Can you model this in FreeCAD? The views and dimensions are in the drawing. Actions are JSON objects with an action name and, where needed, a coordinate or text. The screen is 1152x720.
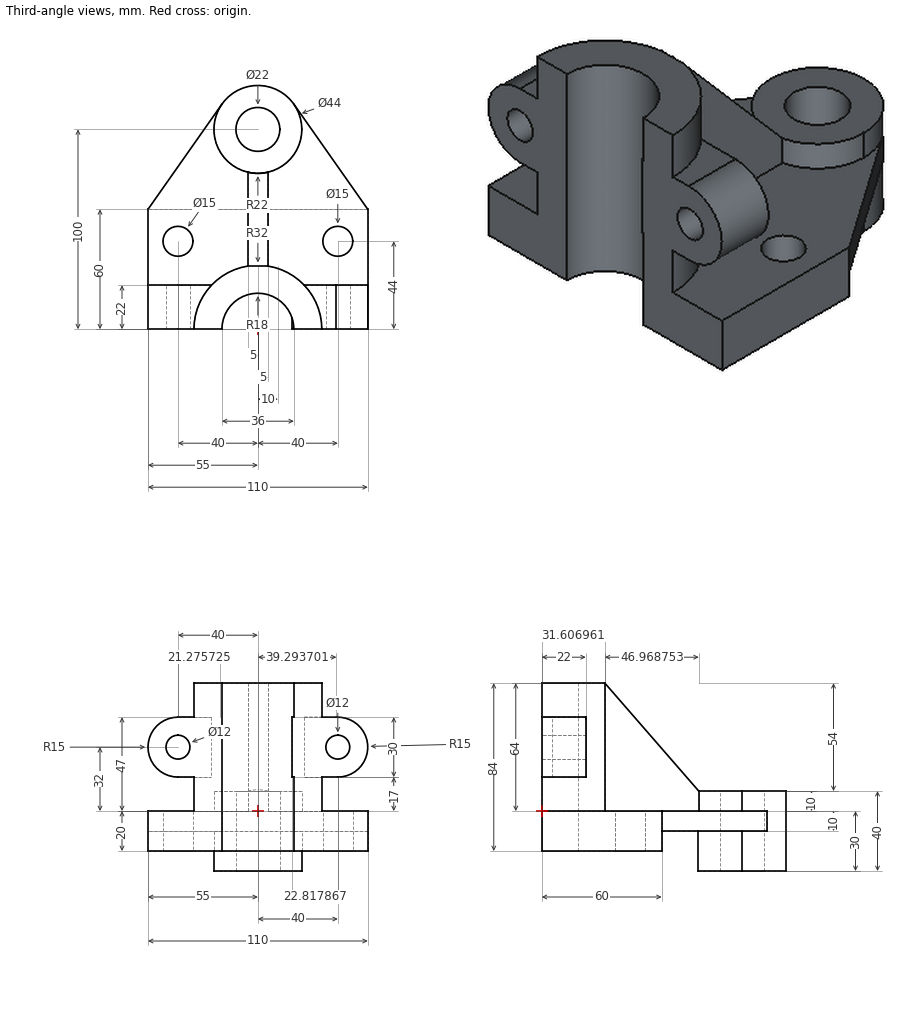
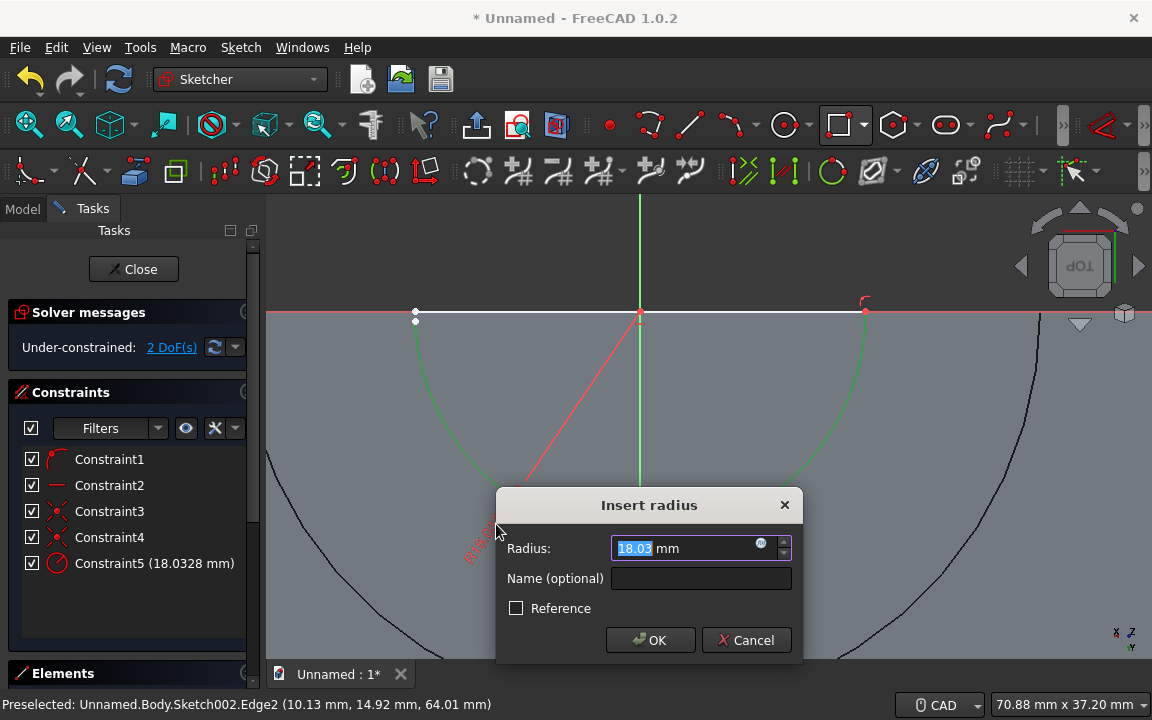
{"action": "type", "text": "18"}
{"action": "key", "text": "Return"}
{"action": "key", "text": "Escape"}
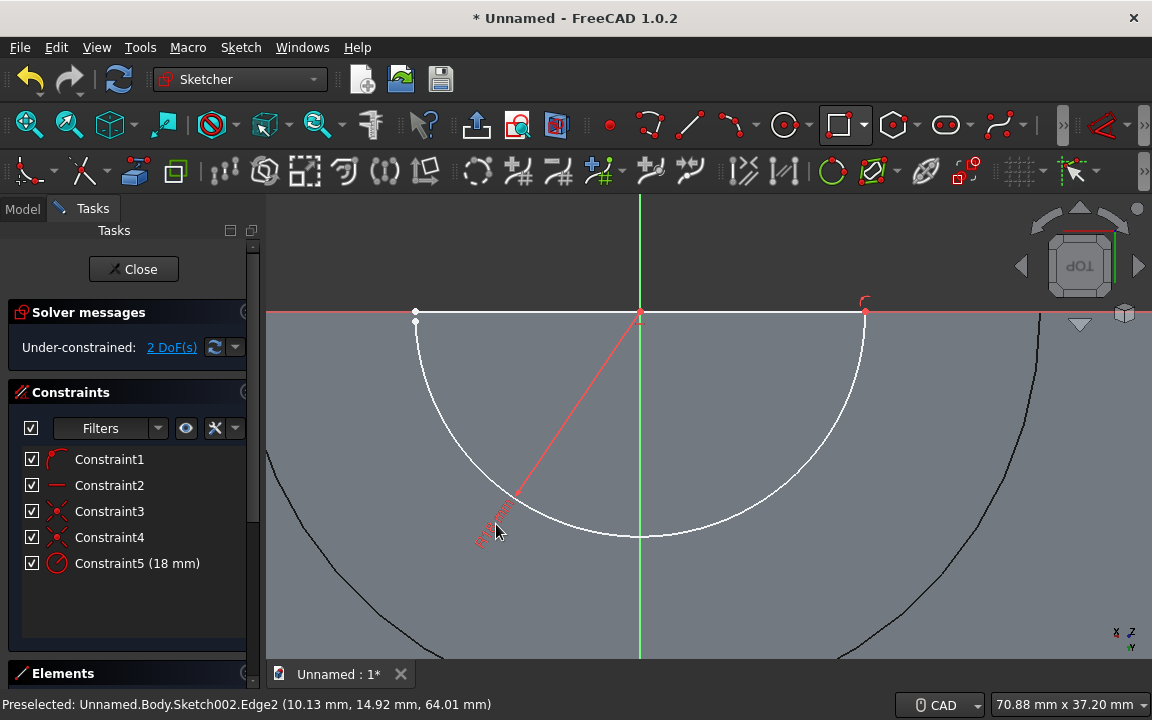
{"action": "left_click", "coordinate": [415, 322]}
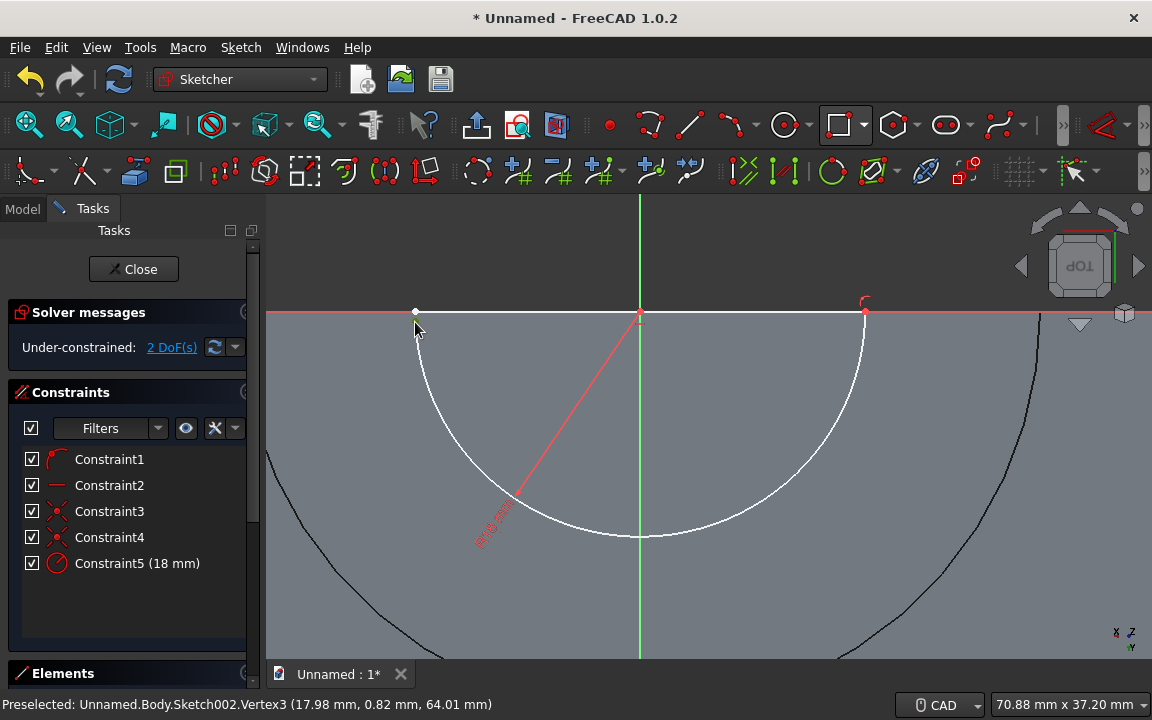
{"action": "left_click", "coordinate": [344, 312]}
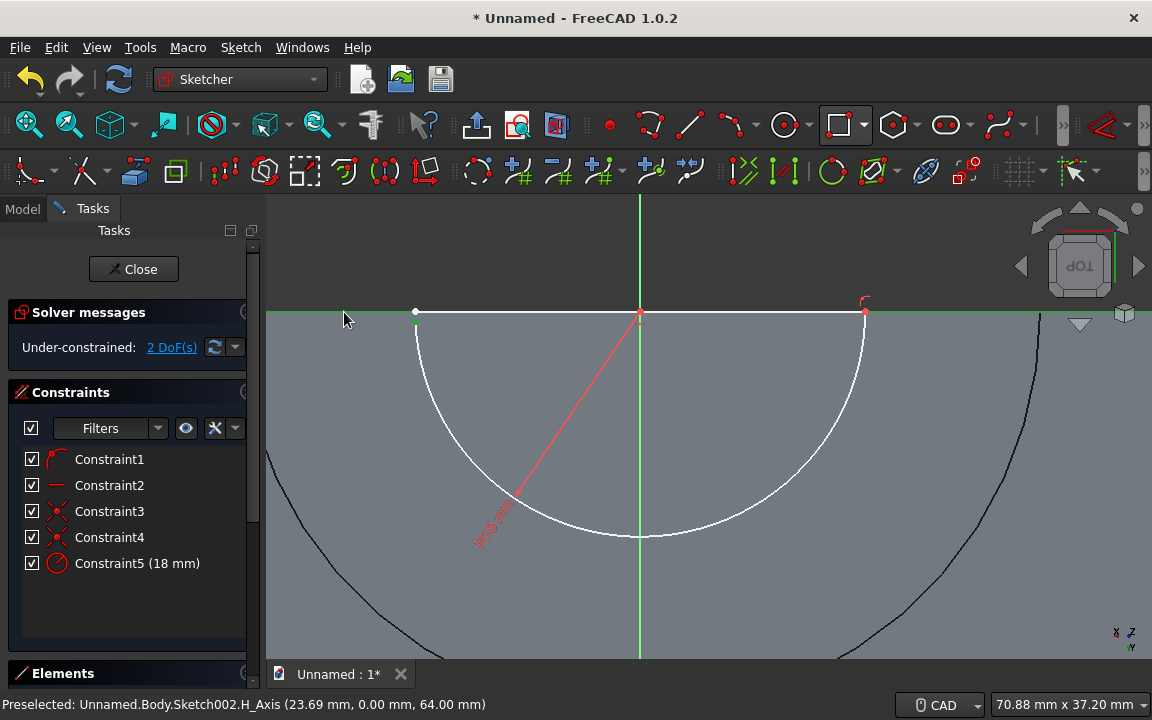
{"action": "key", "text": "c"}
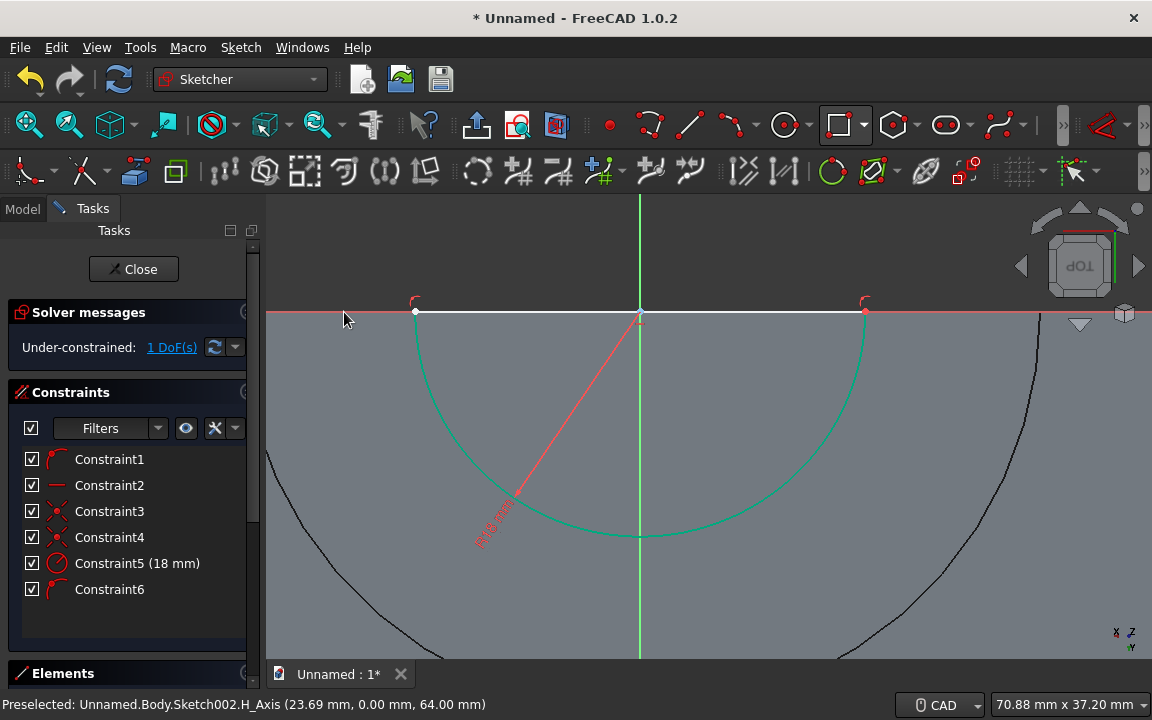
{"action": "left_click", "coordinate": [1102, 126]}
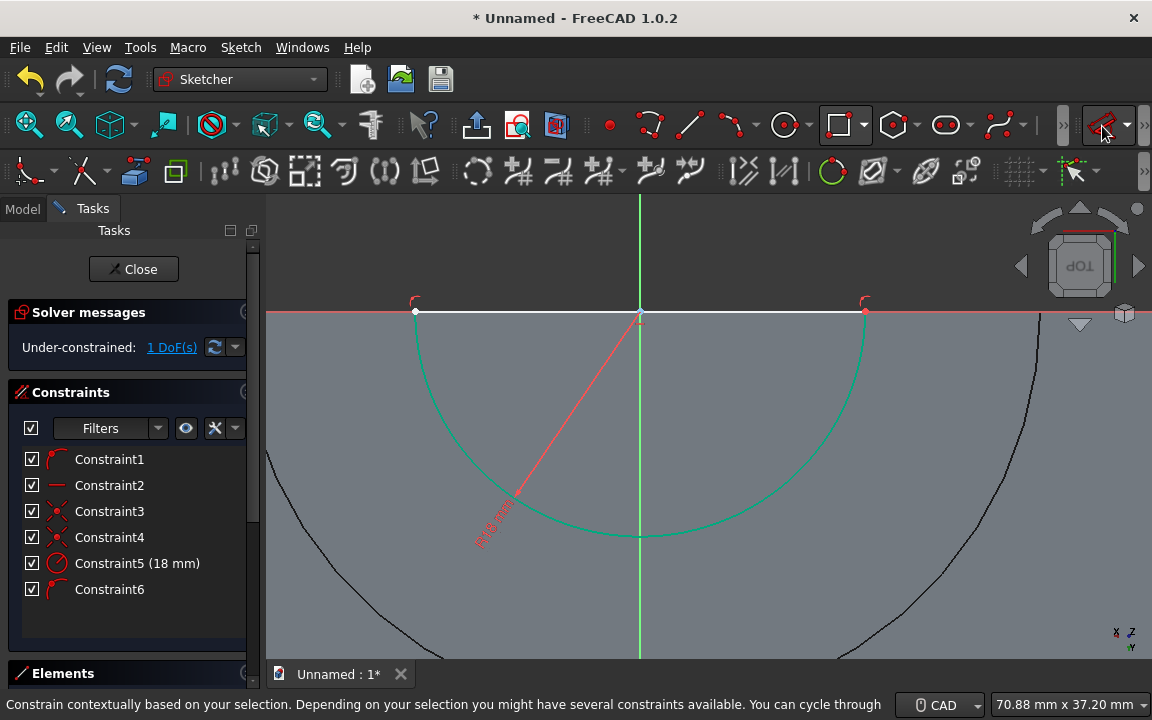
{"action": "left_click", "coordinate": [730, 312]}
{"action": "left_click", "coordinate": [537, 278]}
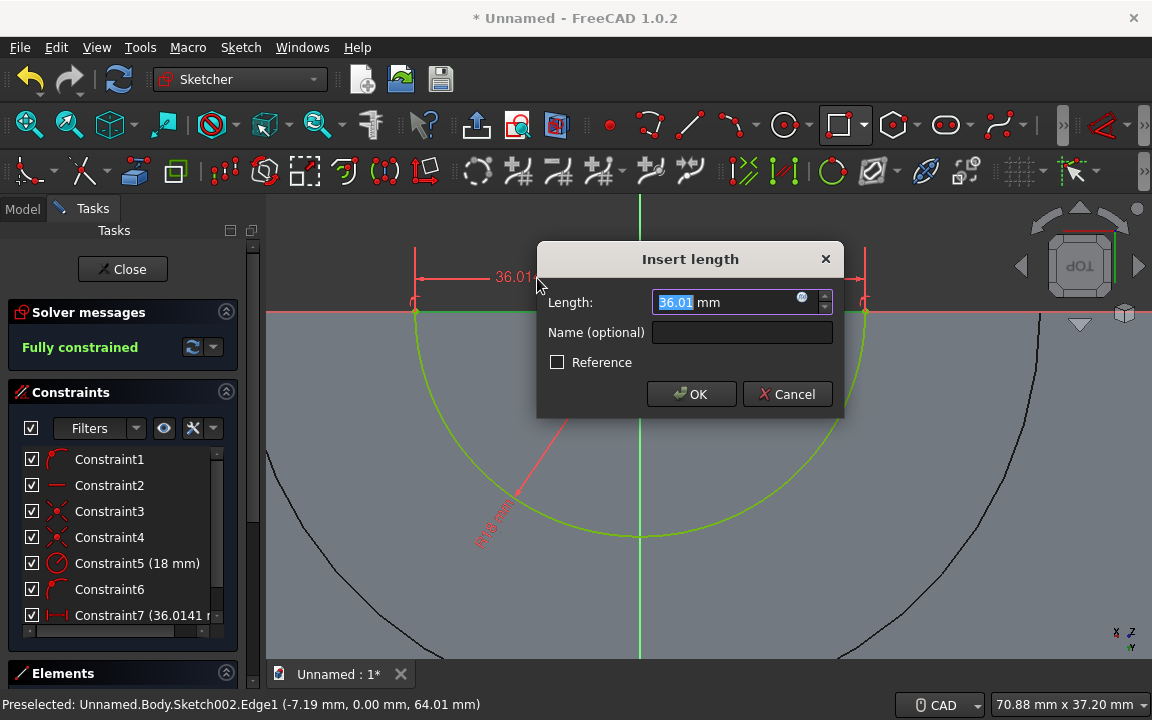
{"action": "type", "text": "36"}
{"action": "key", "text": "Return"}
{"action": "key", "text": "Escape"}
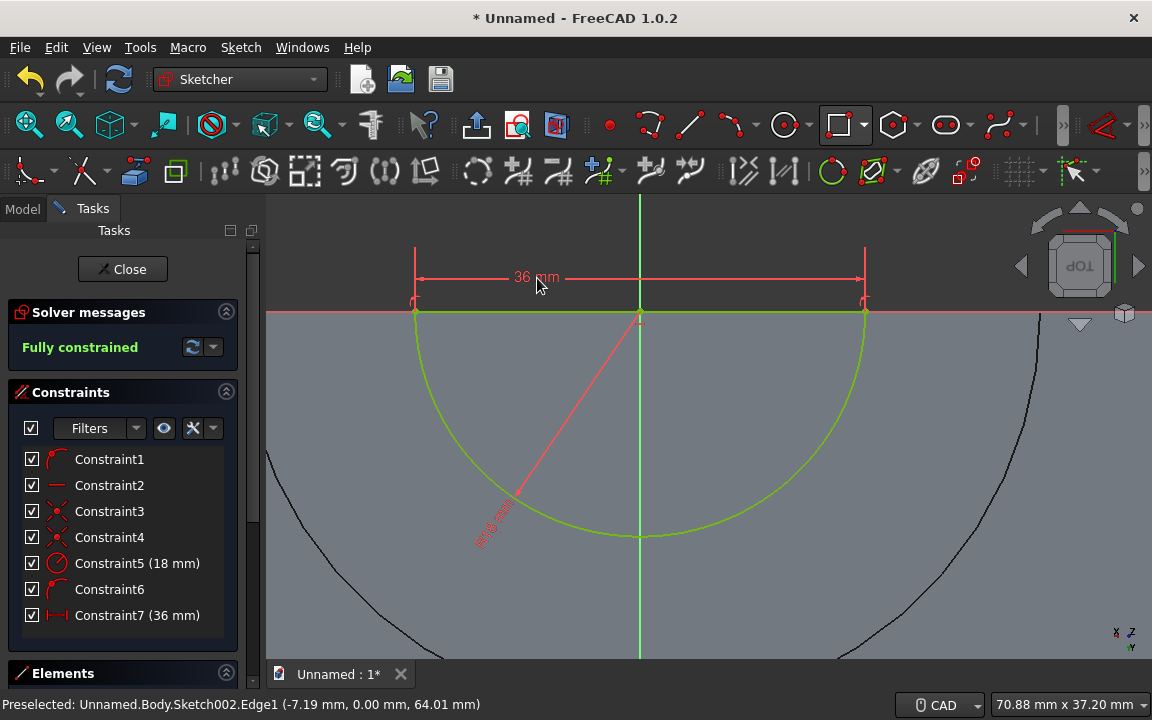
{"action": "left_click", "coordinate": [123, 269]}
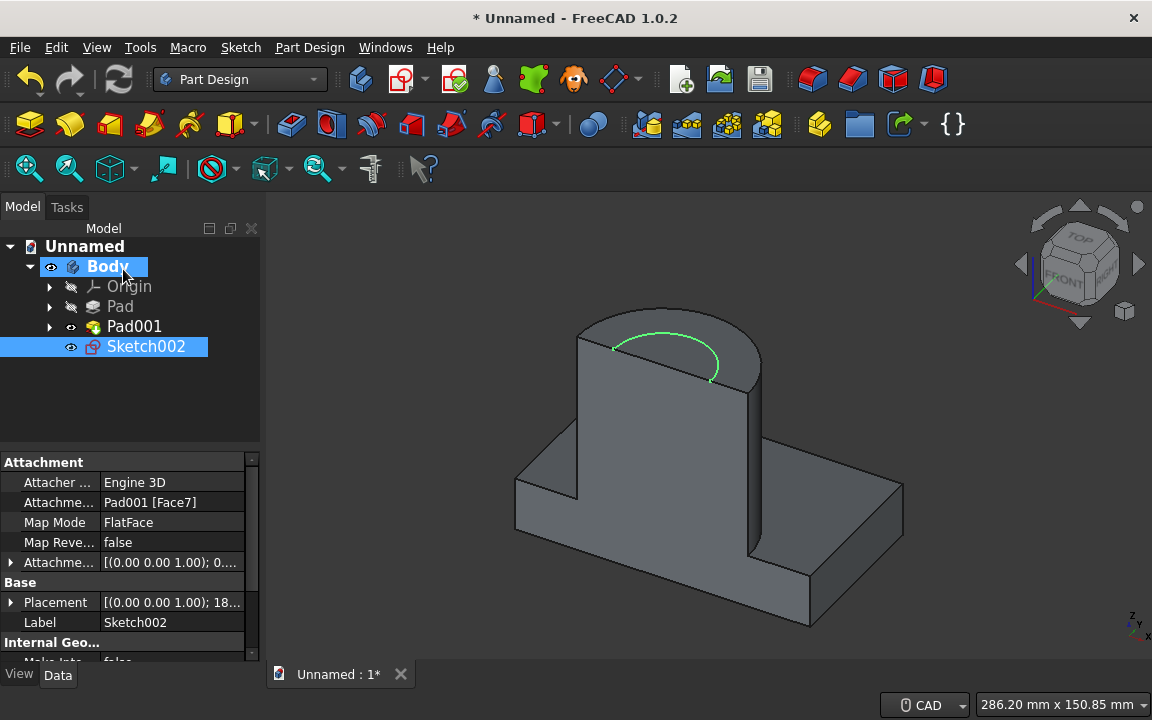
{"action": "left_click", "coordinate": [292, 124]}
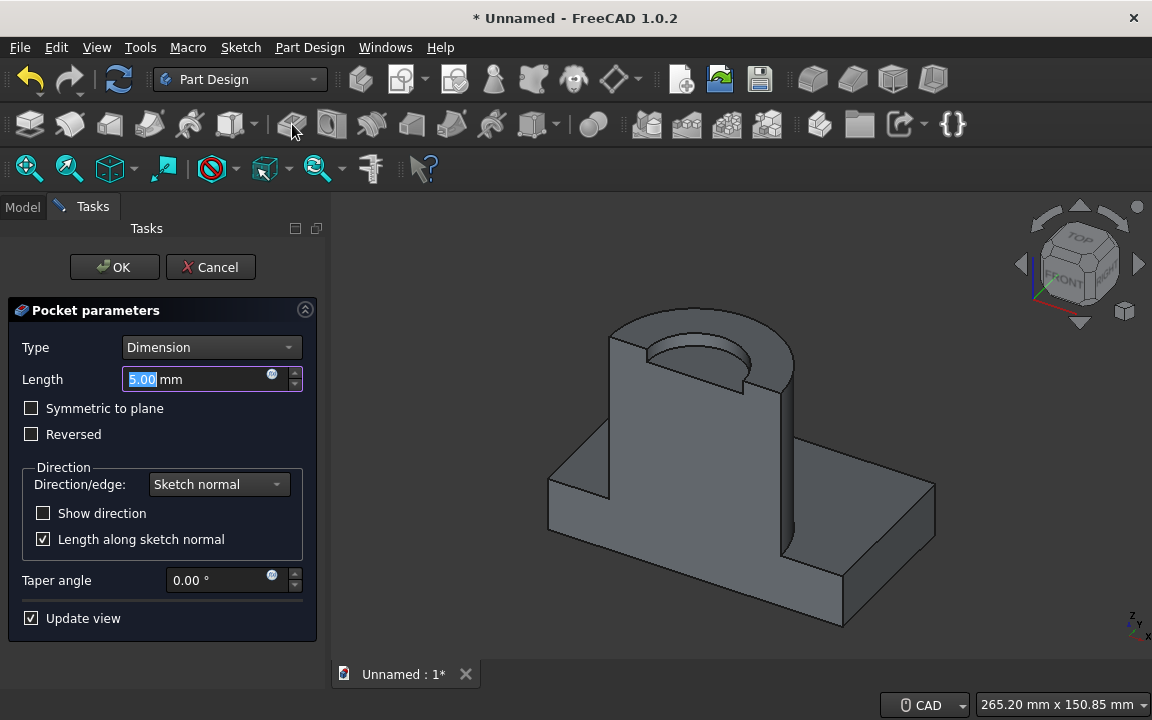
{"action": "type", "text": "84"}
{"action": "key", "text": "Tab"}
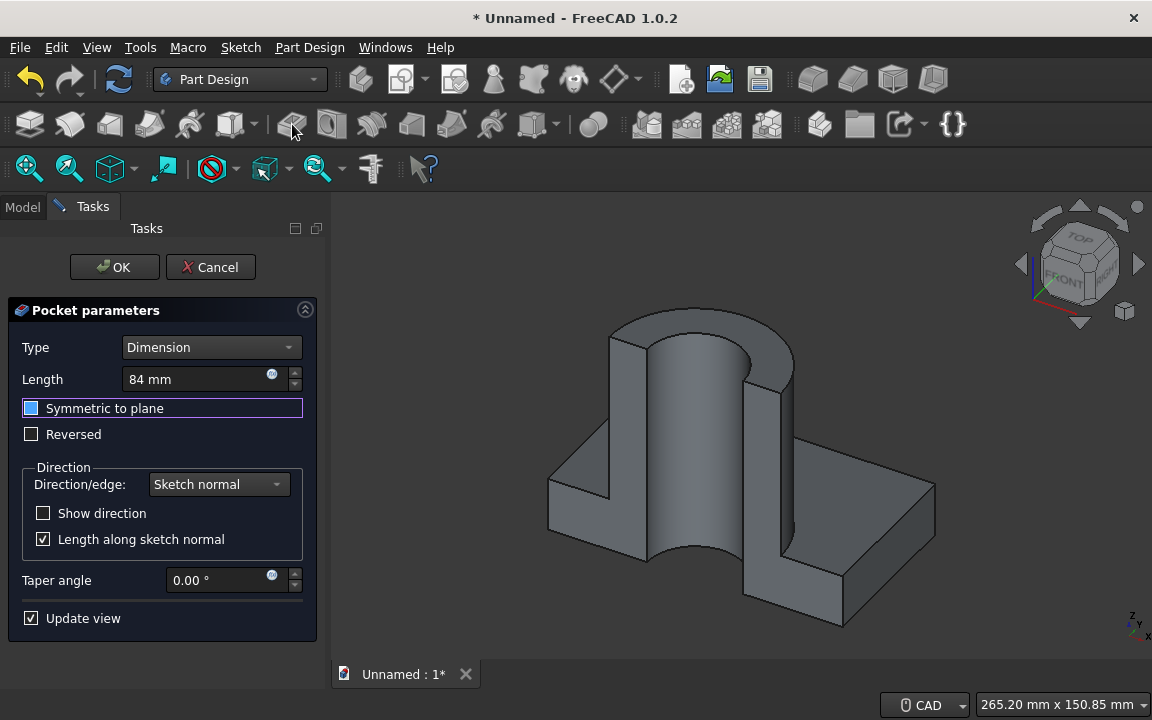
{"action": "left_click", "coordinate": [115, 267]}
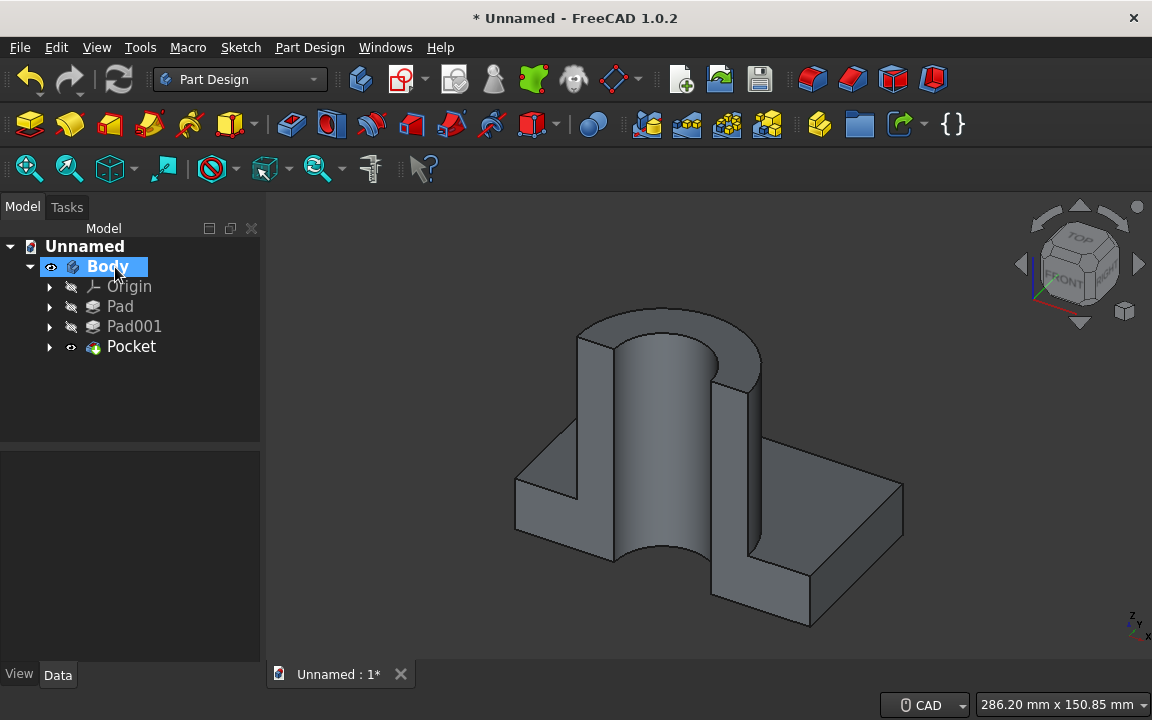
{"action": "left_click", "coordinate": [593, 508]}